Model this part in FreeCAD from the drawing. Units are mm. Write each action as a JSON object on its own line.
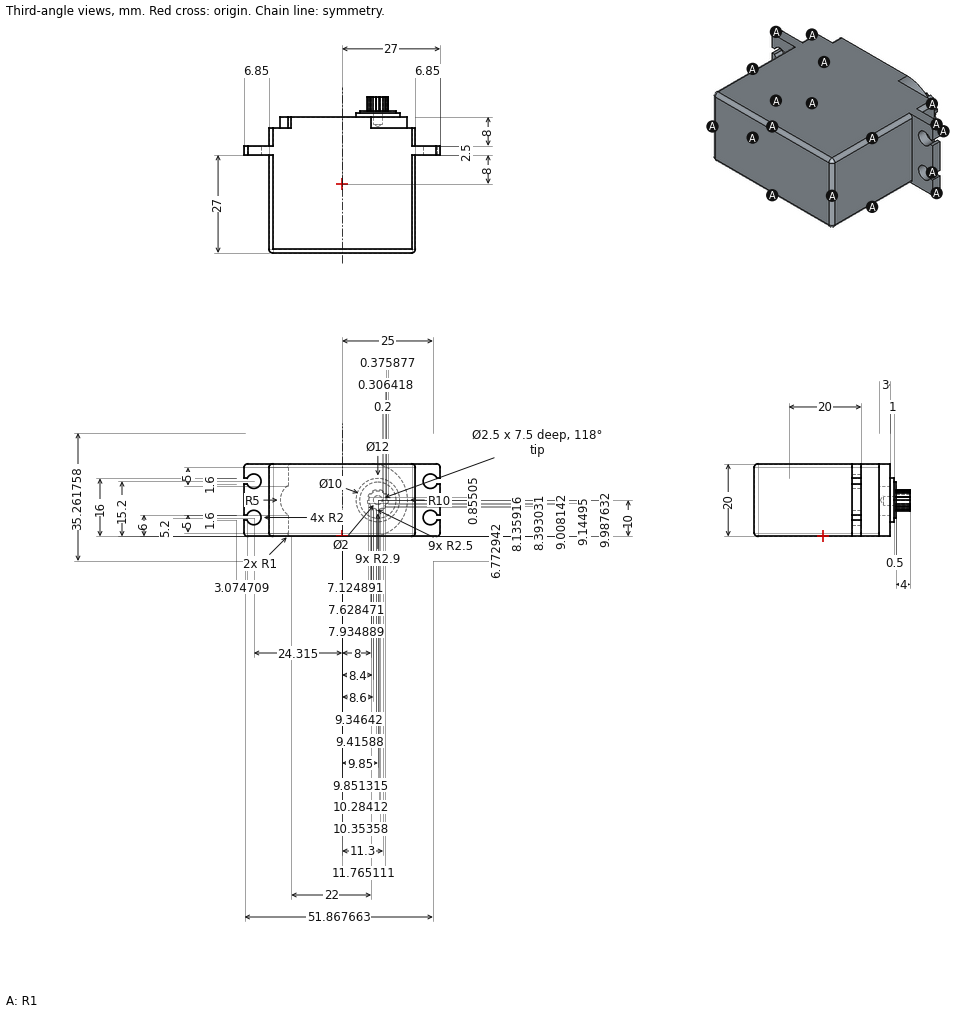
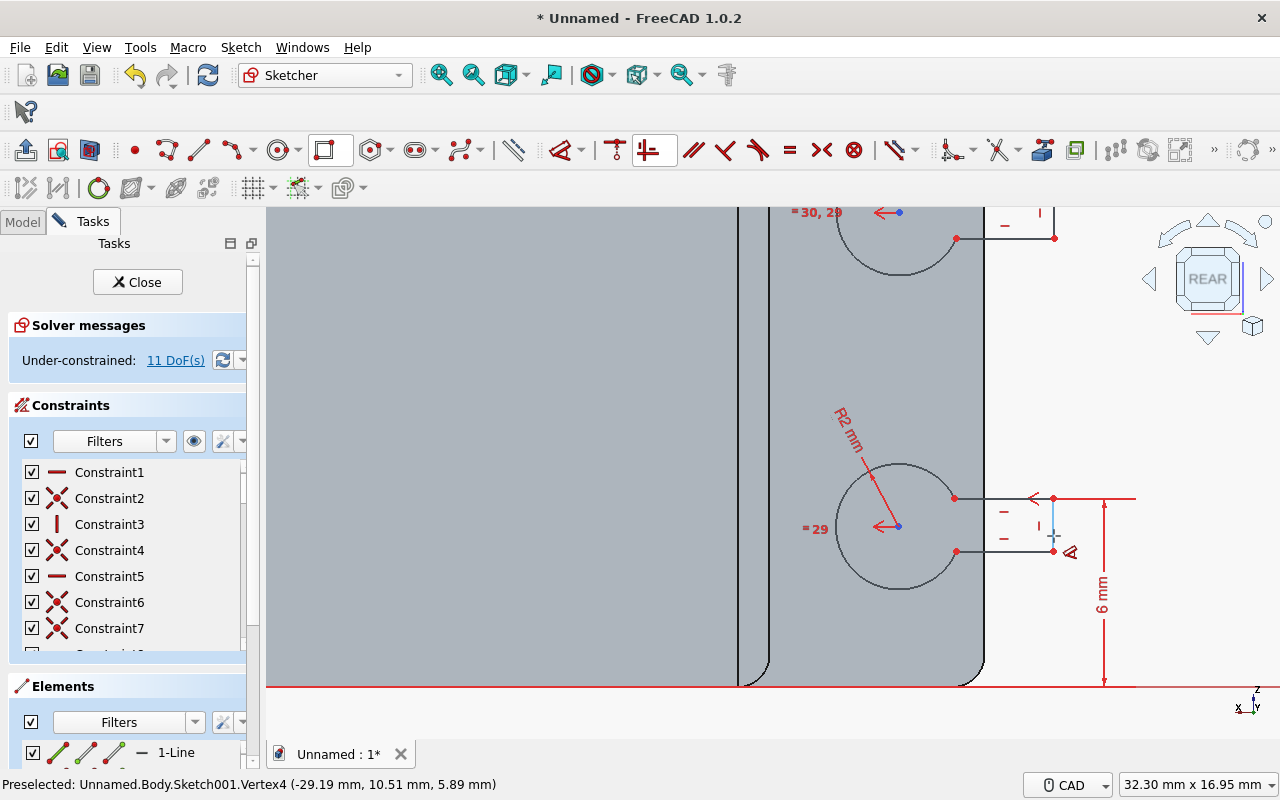
{"action": "left_click", "coordinate": [1053, 536]}
{"action": "left_click", "coordinate": [1087, 525]}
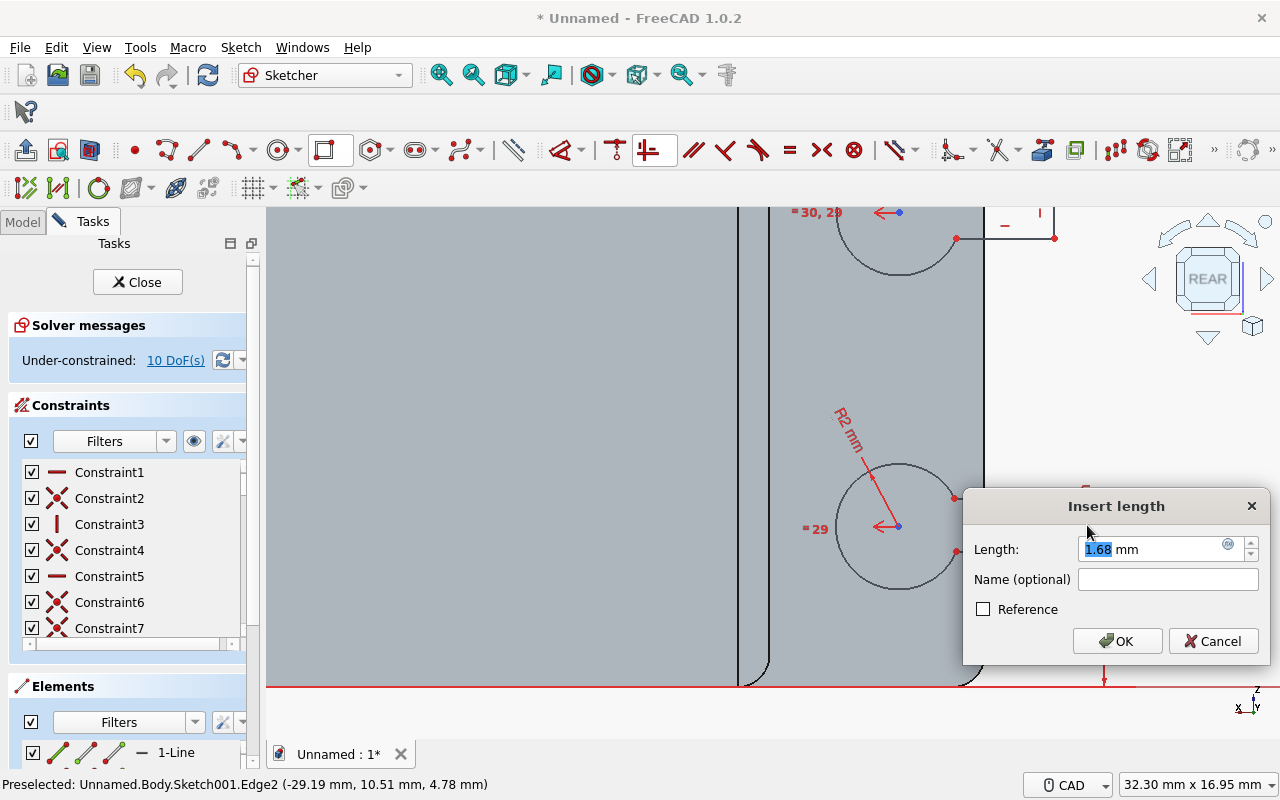
{"action": "type", "text": "1.6"}
{"action": "key", "text": "Return"}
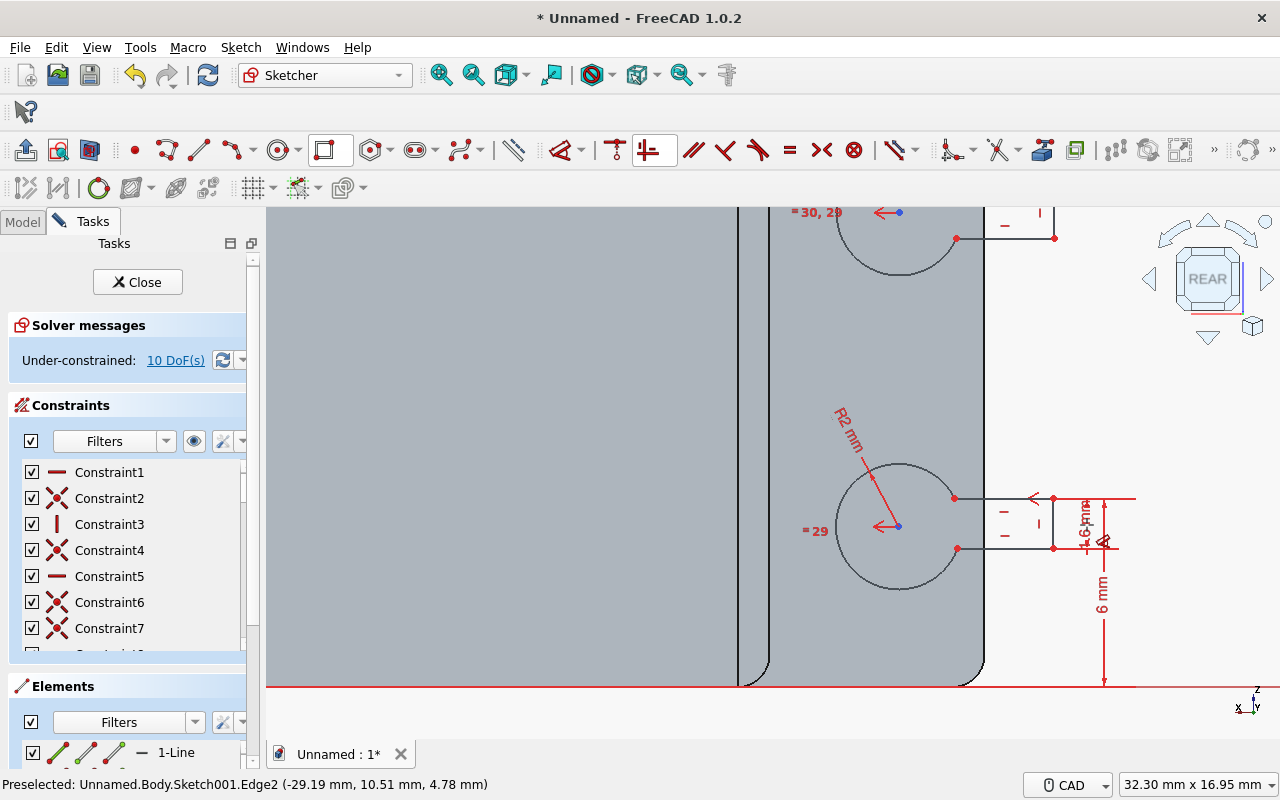
{"action": "scroll", "coordinate": [949, 489], "scroll_direction": "down", "scroll_amount": 6}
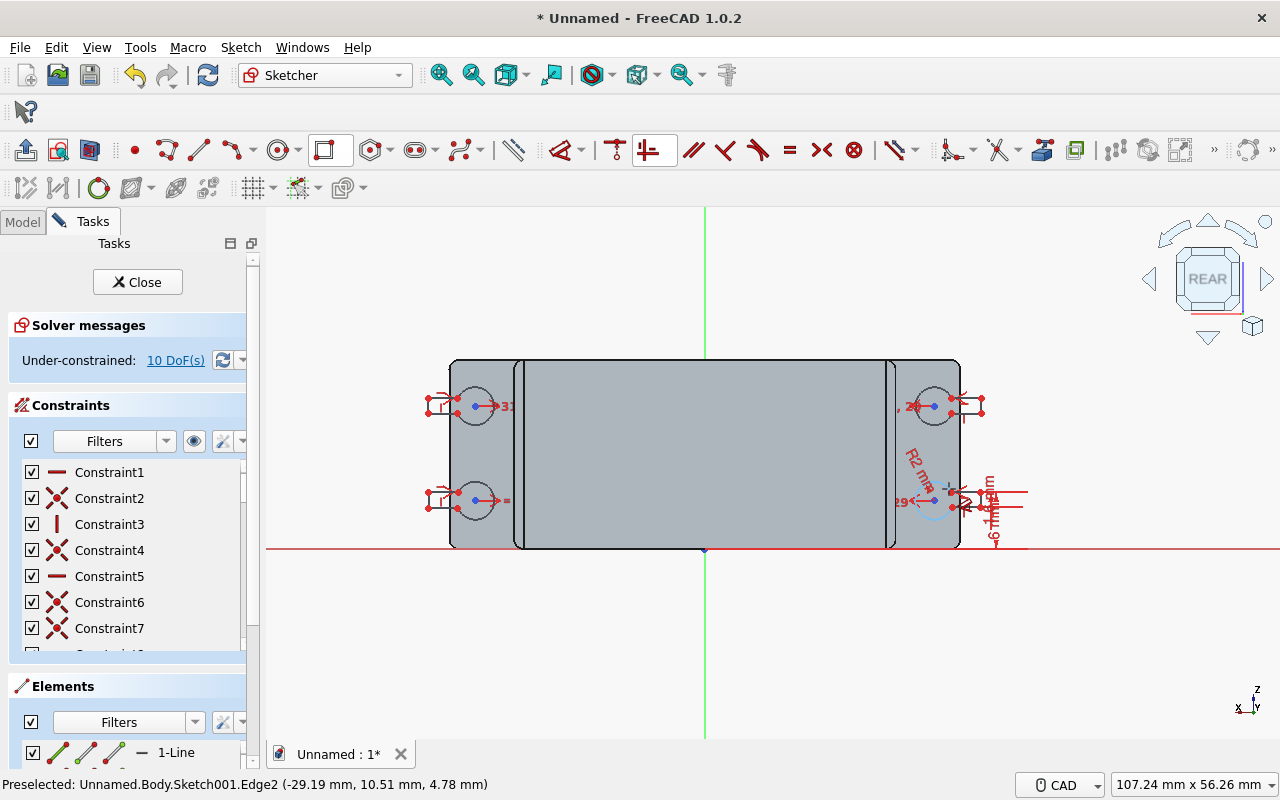
{"action": "scroll", "coordinate": [981, 409], "scroll_direction": "up", "scroll_amount": 6}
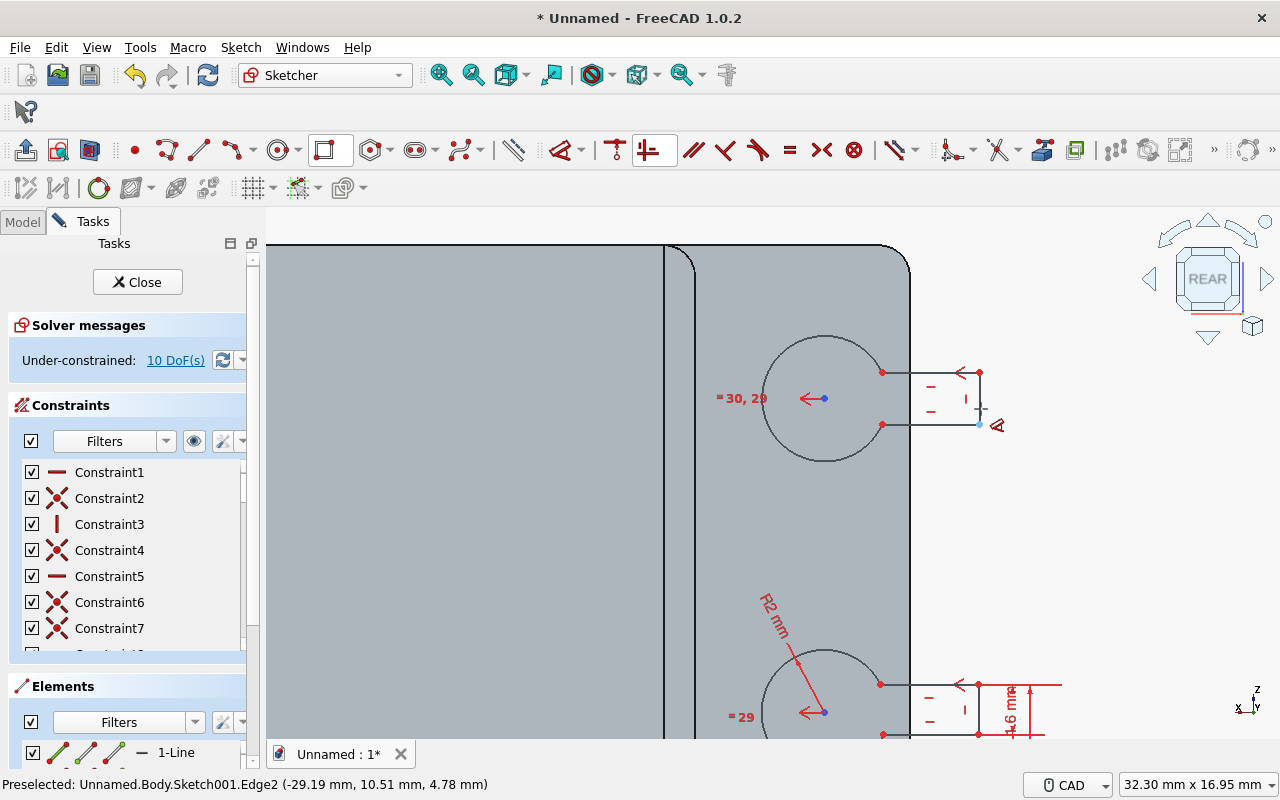
{"action": "left_click", "coordinate": [980, 409]}
{"action": "left_click", "coordinate": [1014, 399]}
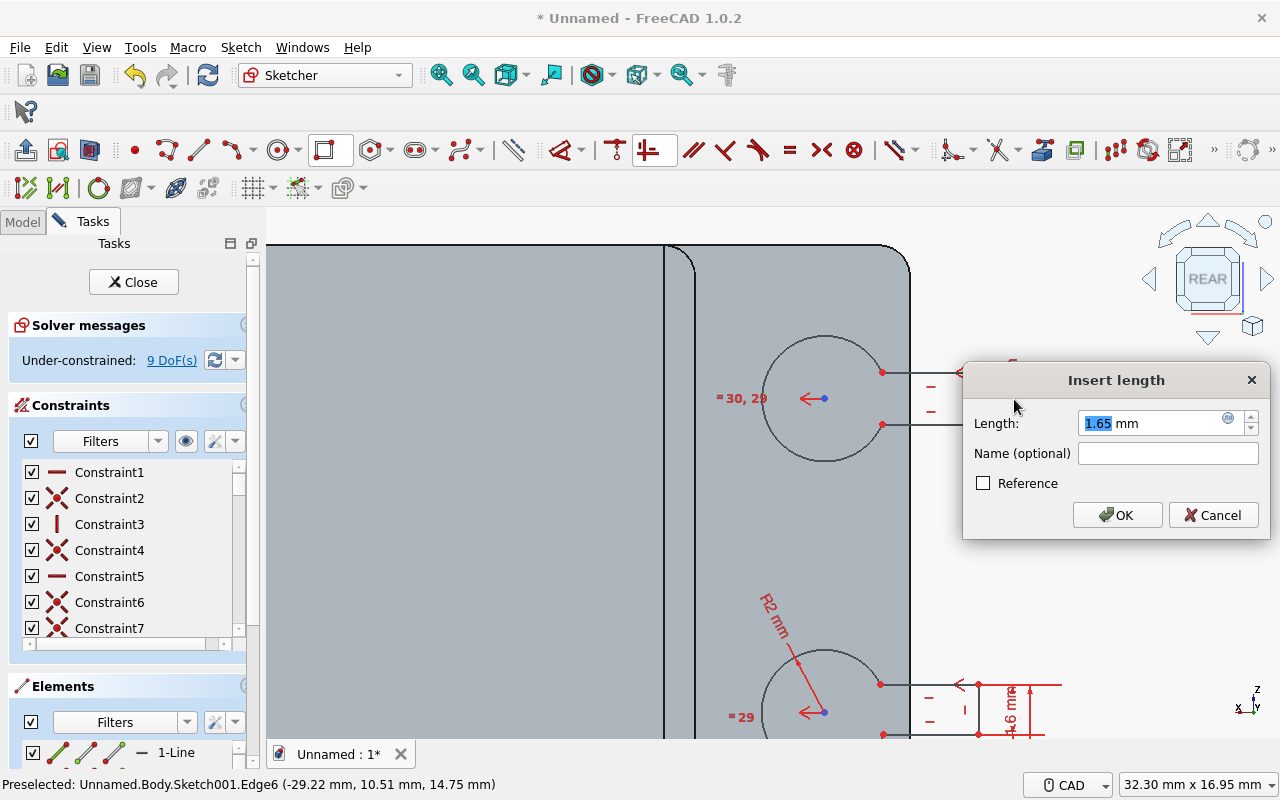
{"action": "type", "text": "1.6"}
{"action": "key", "text": "Return"}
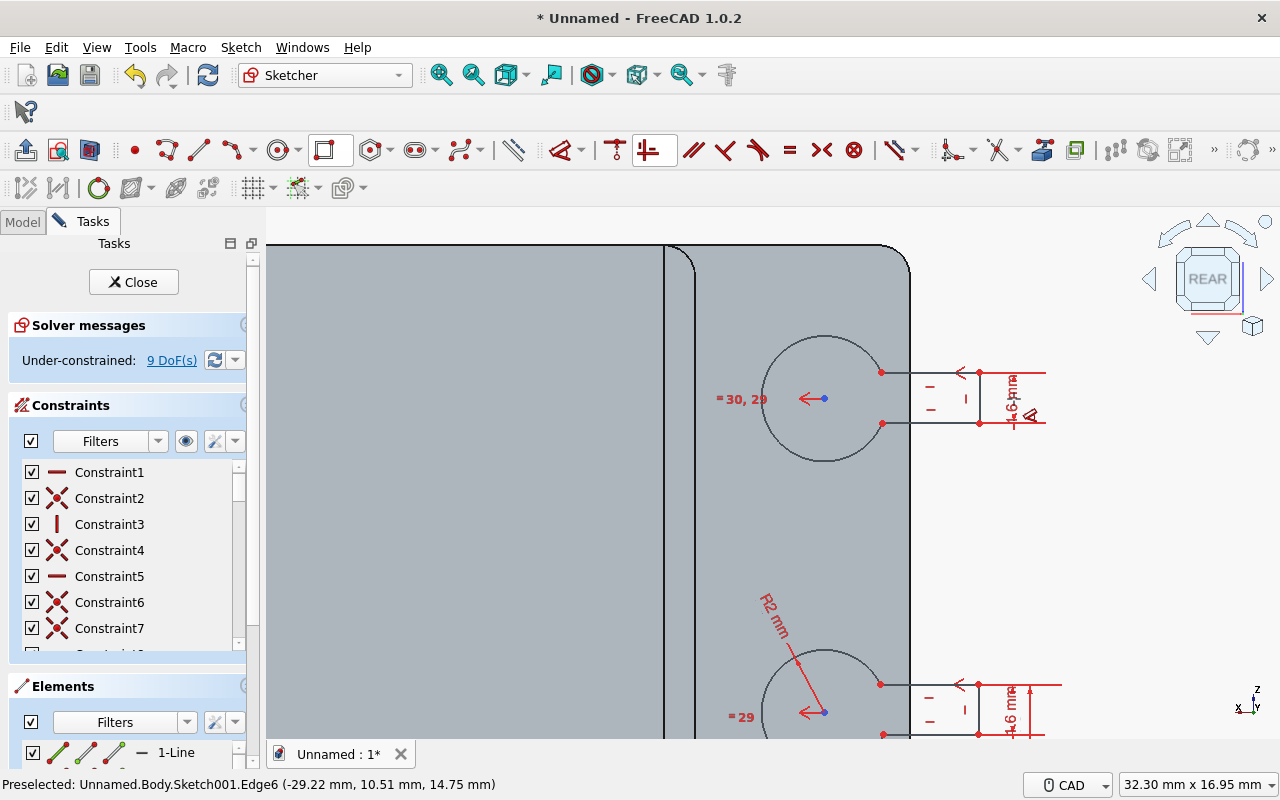
{"action": "scroll", "coordinate": [981, 409], "scroll_direction": "down", "scroll_amount": 6}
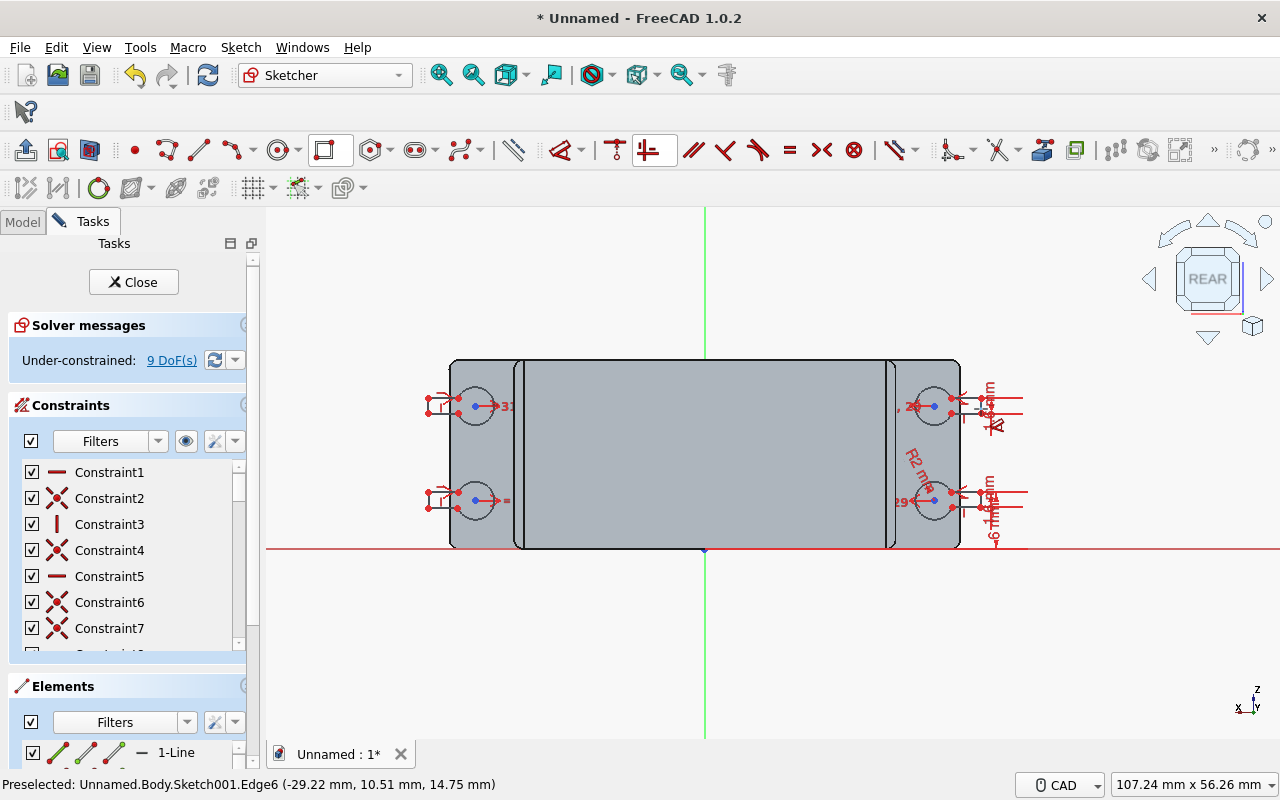
{"action": "scroll", "coordinate": [428, 403], "scroll_direction": "up", "scroll_amount": 6}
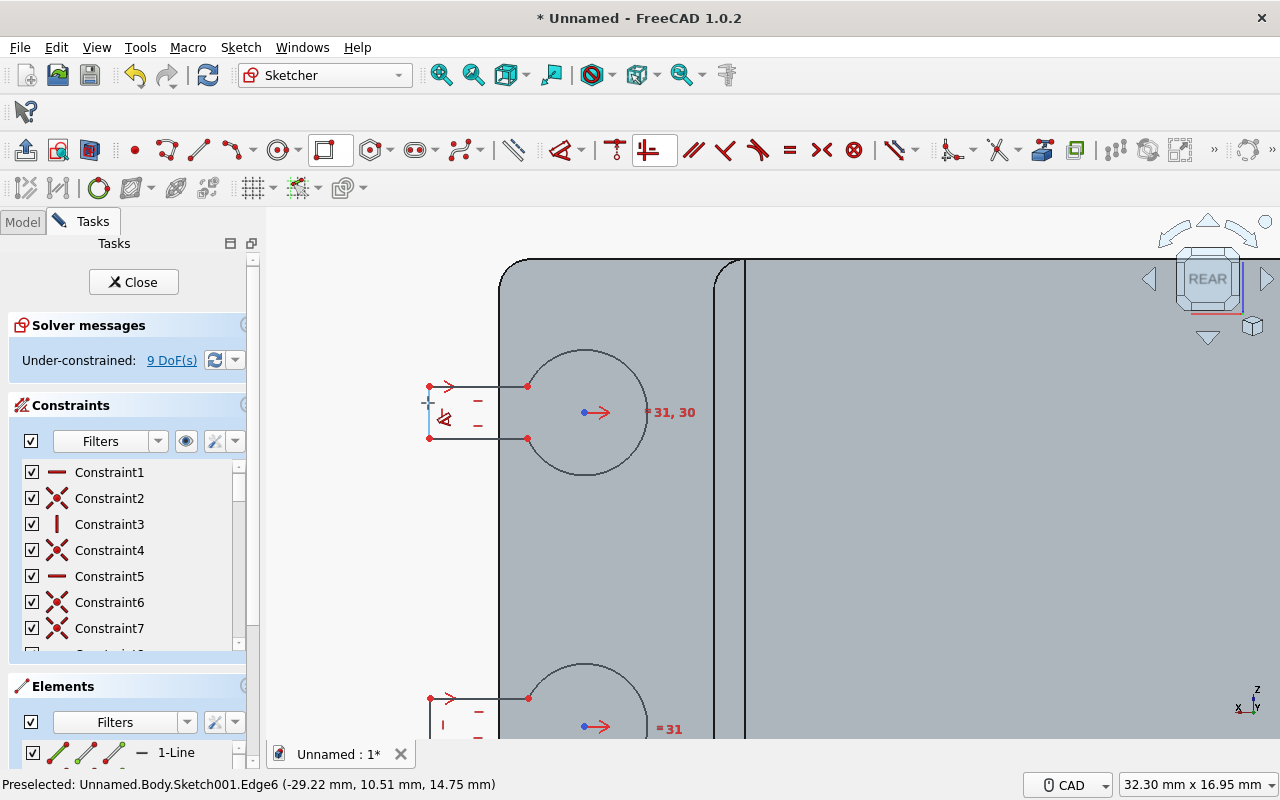
{"action": "left_click", "coordinate": [429, 402]}
{"action": "left_click", "coordinate": [395, 413]}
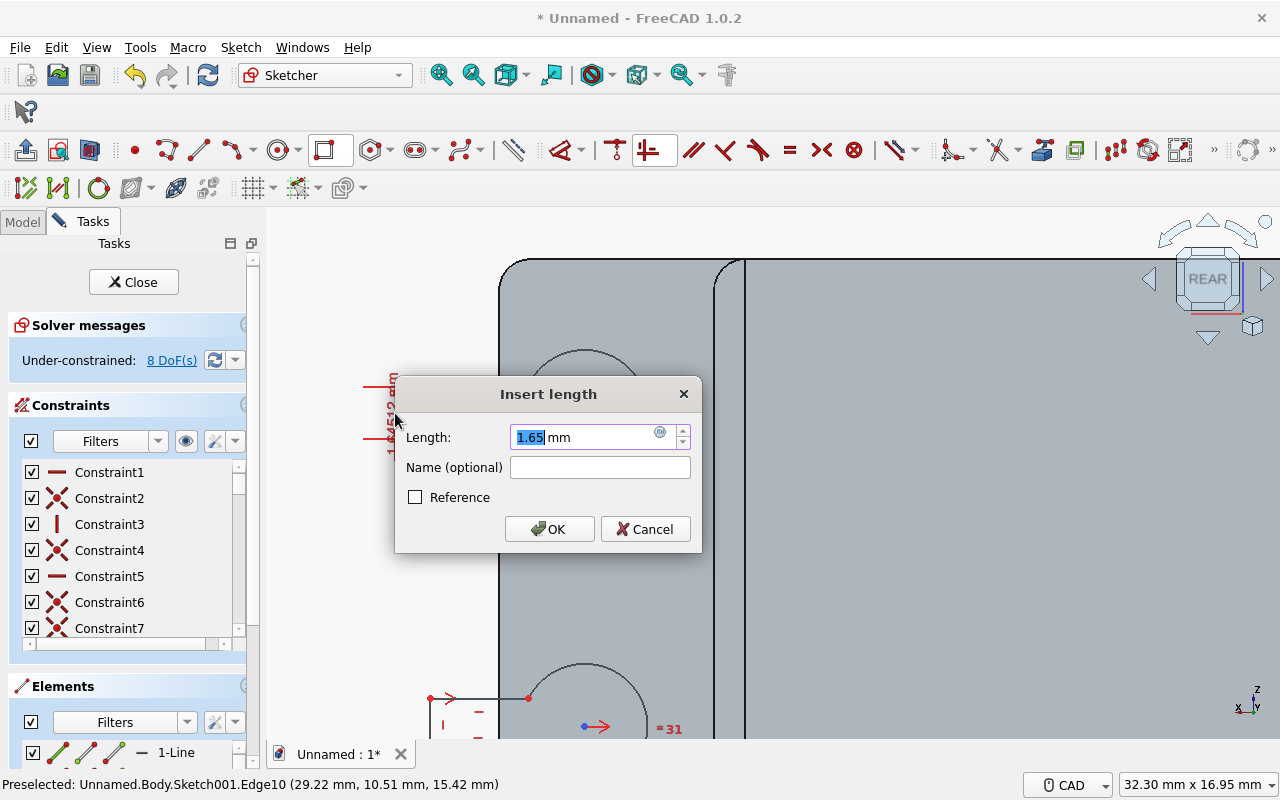
{"action": "type", "text": "1.6"}
{"action": "key", "text": "Return"}